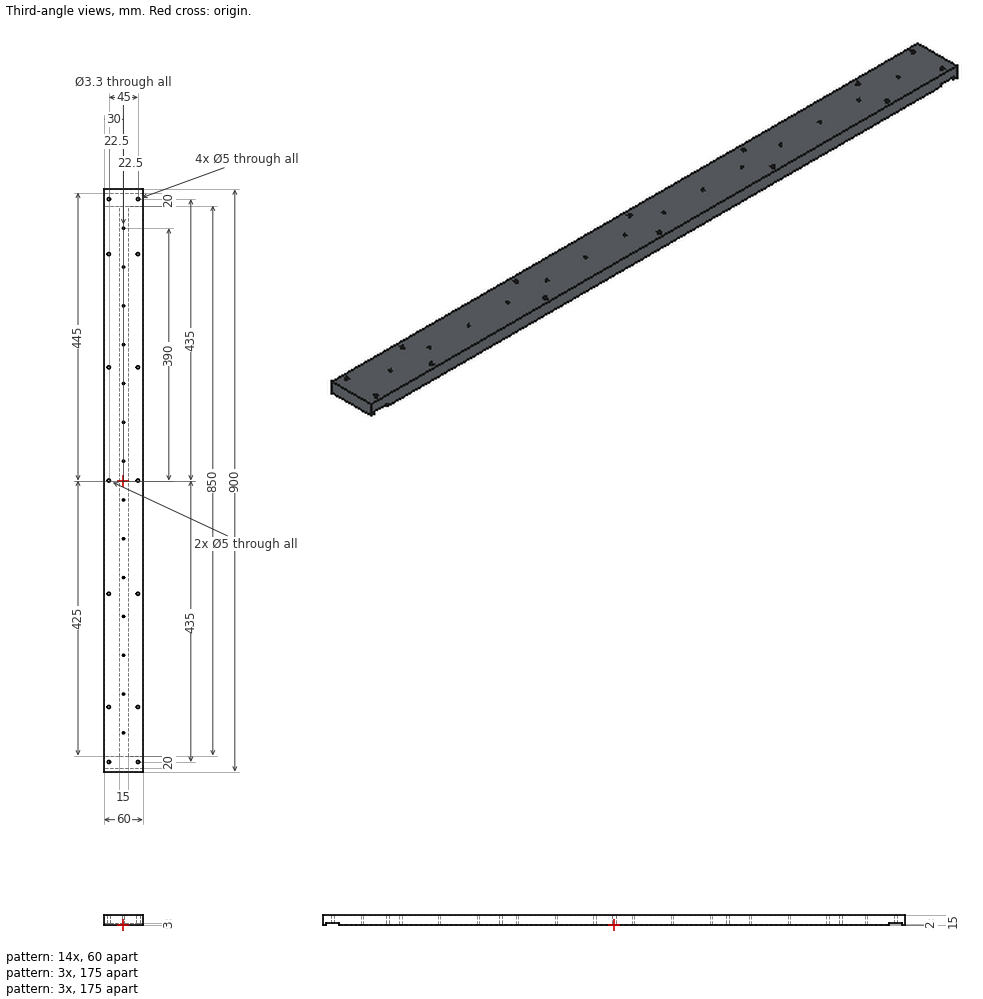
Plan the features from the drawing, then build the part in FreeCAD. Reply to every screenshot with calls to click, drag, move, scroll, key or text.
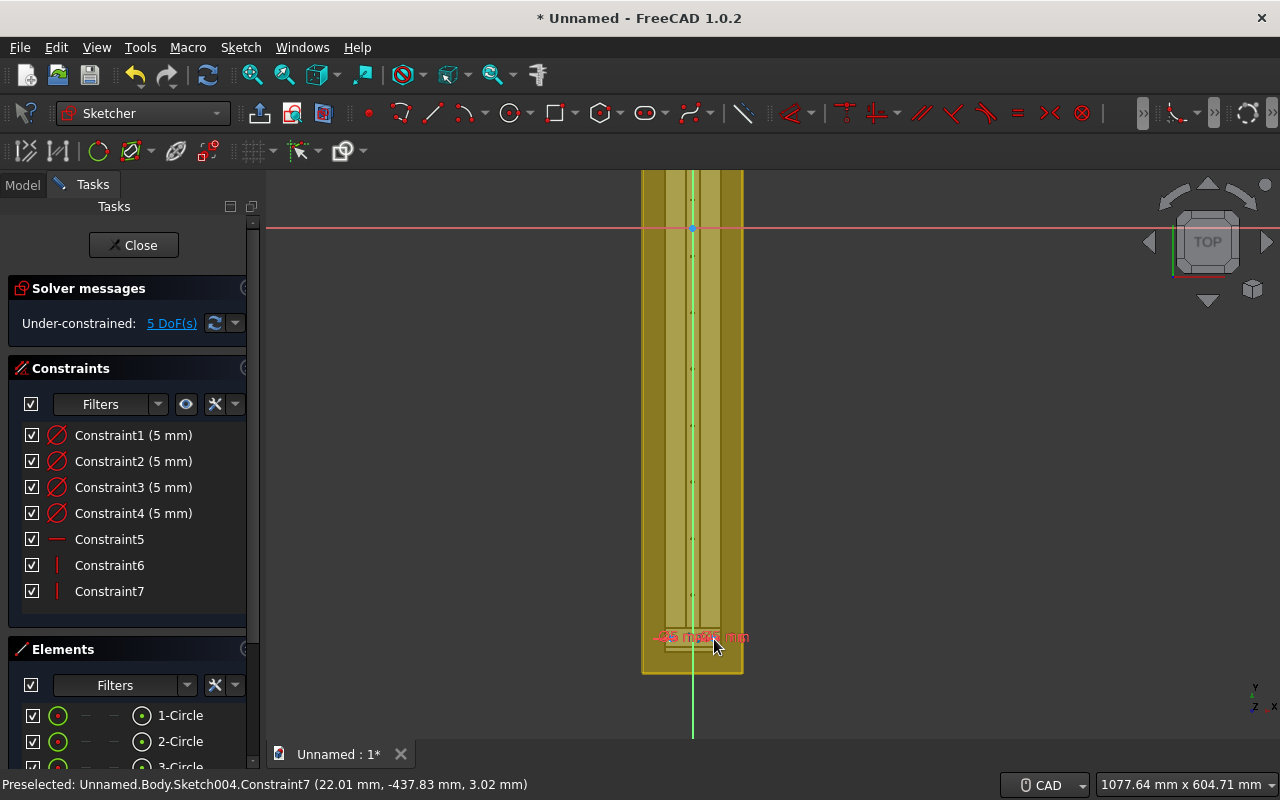
click(713, 639)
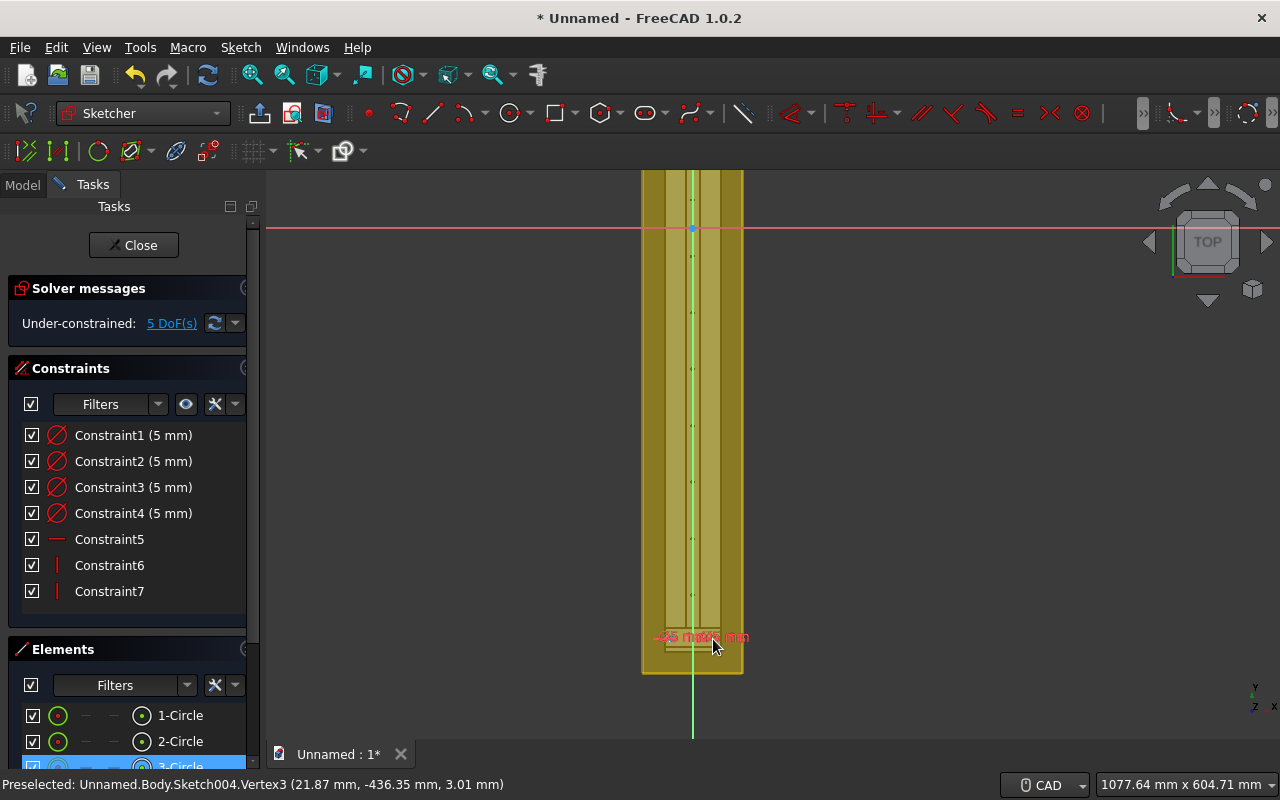
click(671, 639)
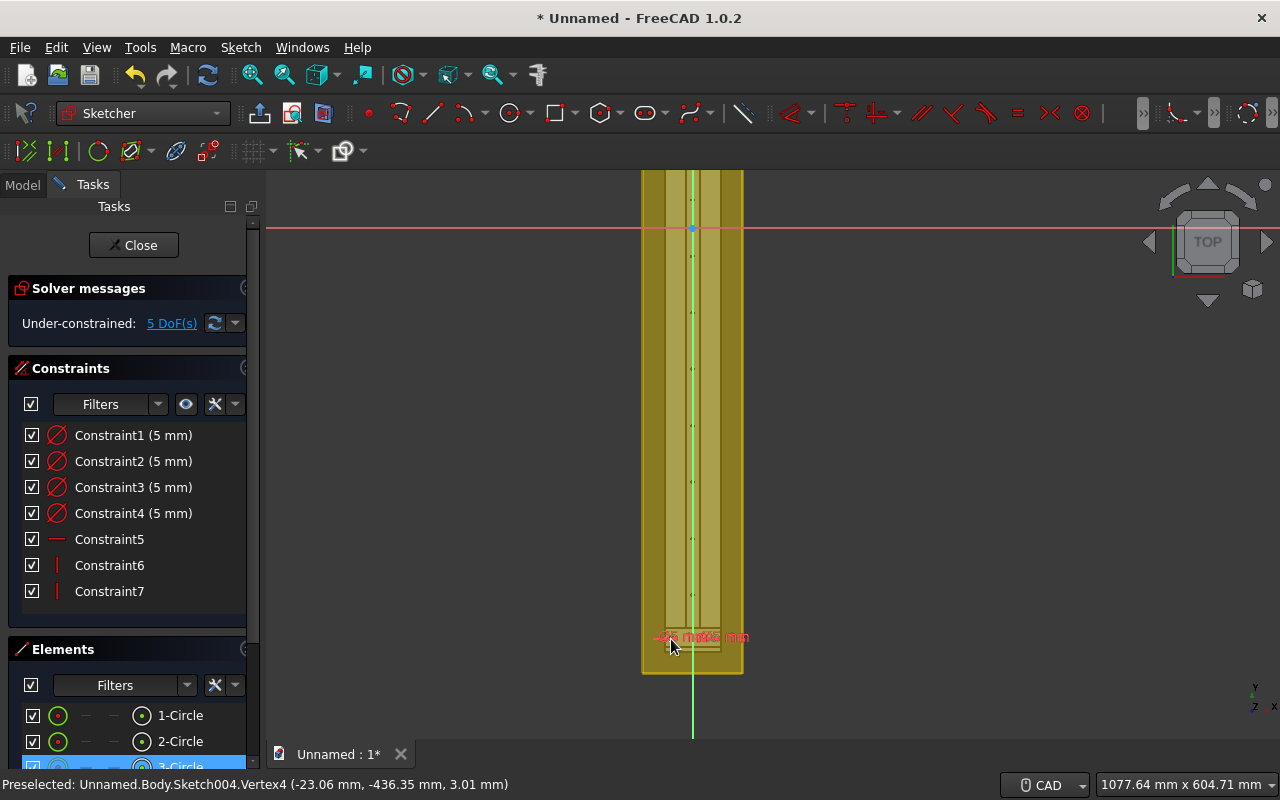
click(900, 114)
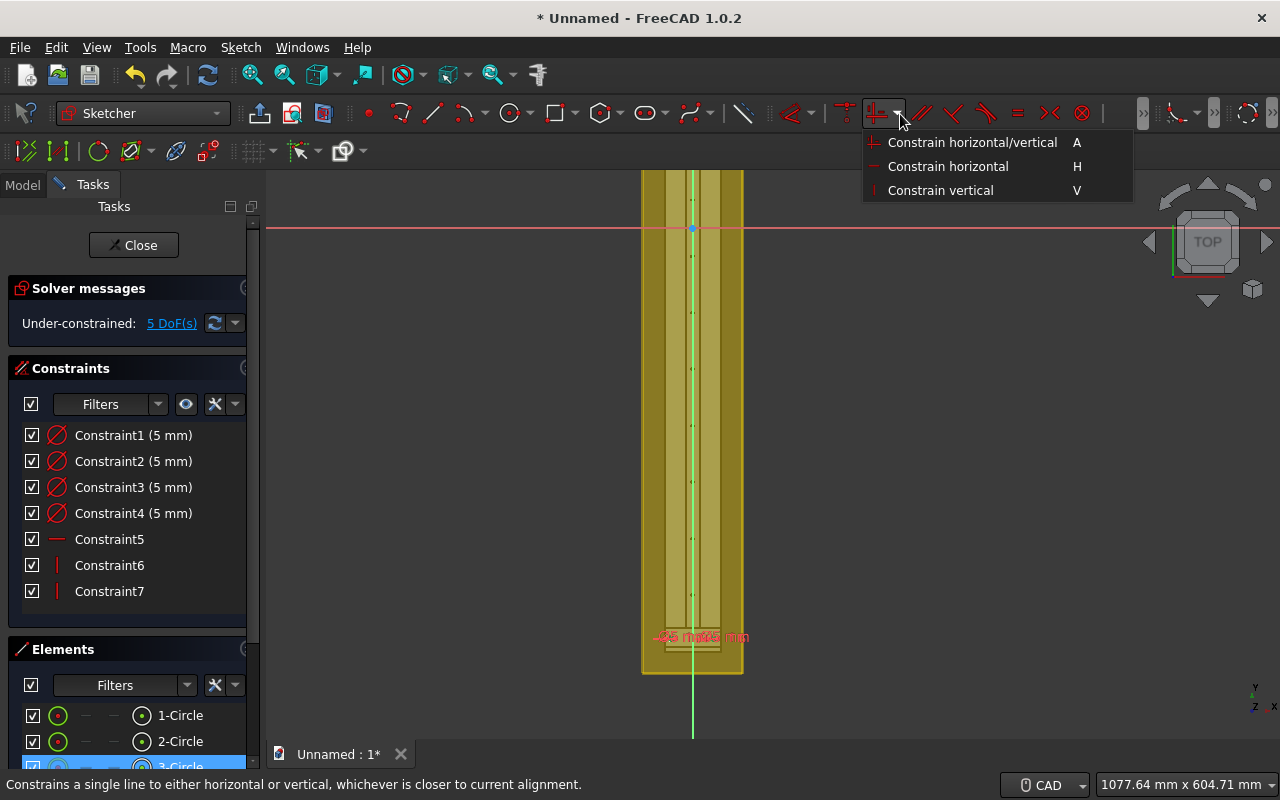
click(998, 166)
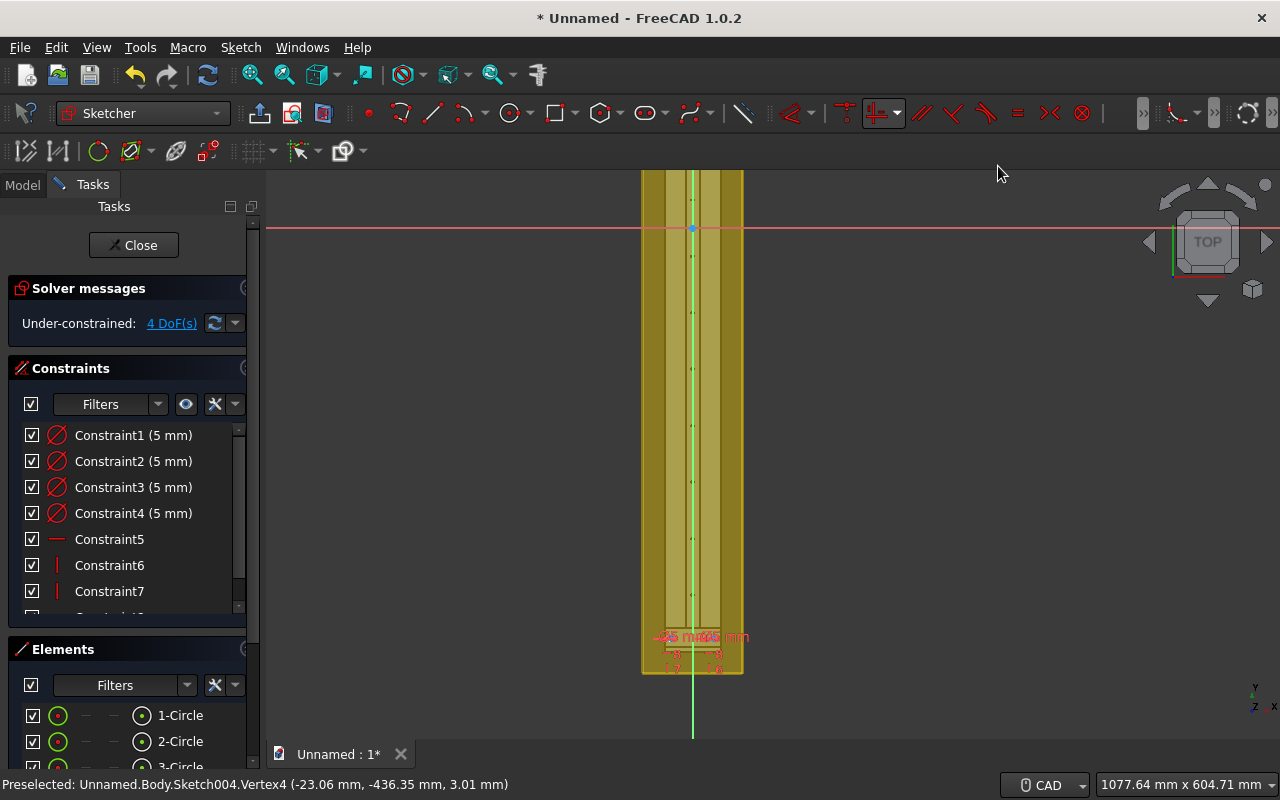
key(d)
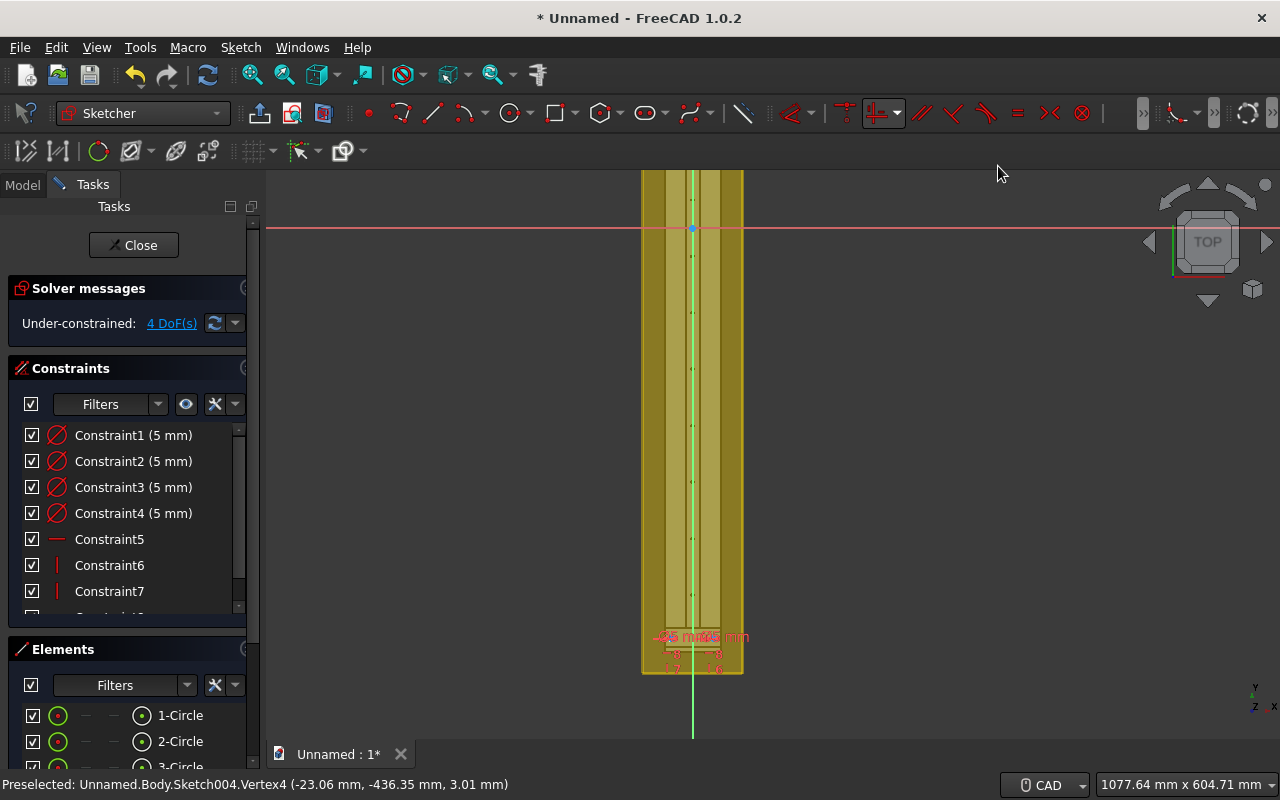
scroll(714, 639, down, 4)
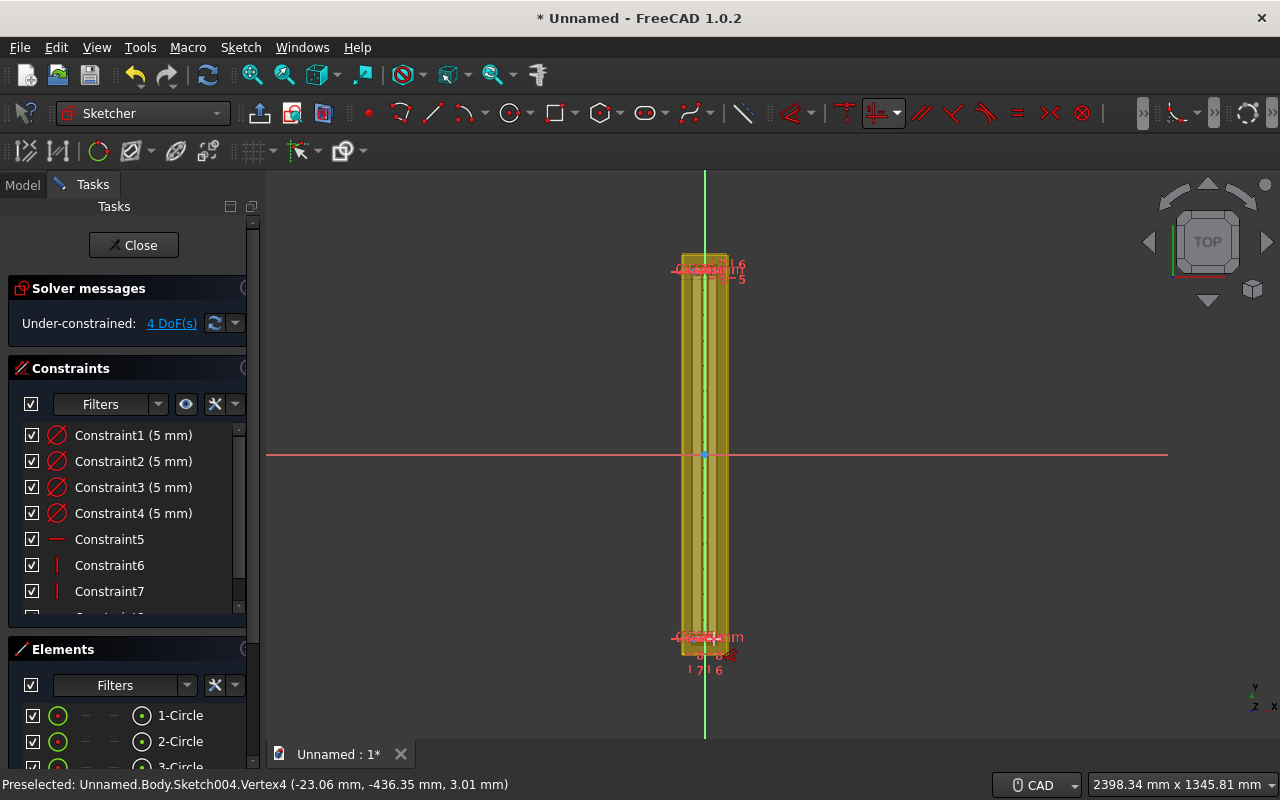
click(714, 272)
click(748, 363)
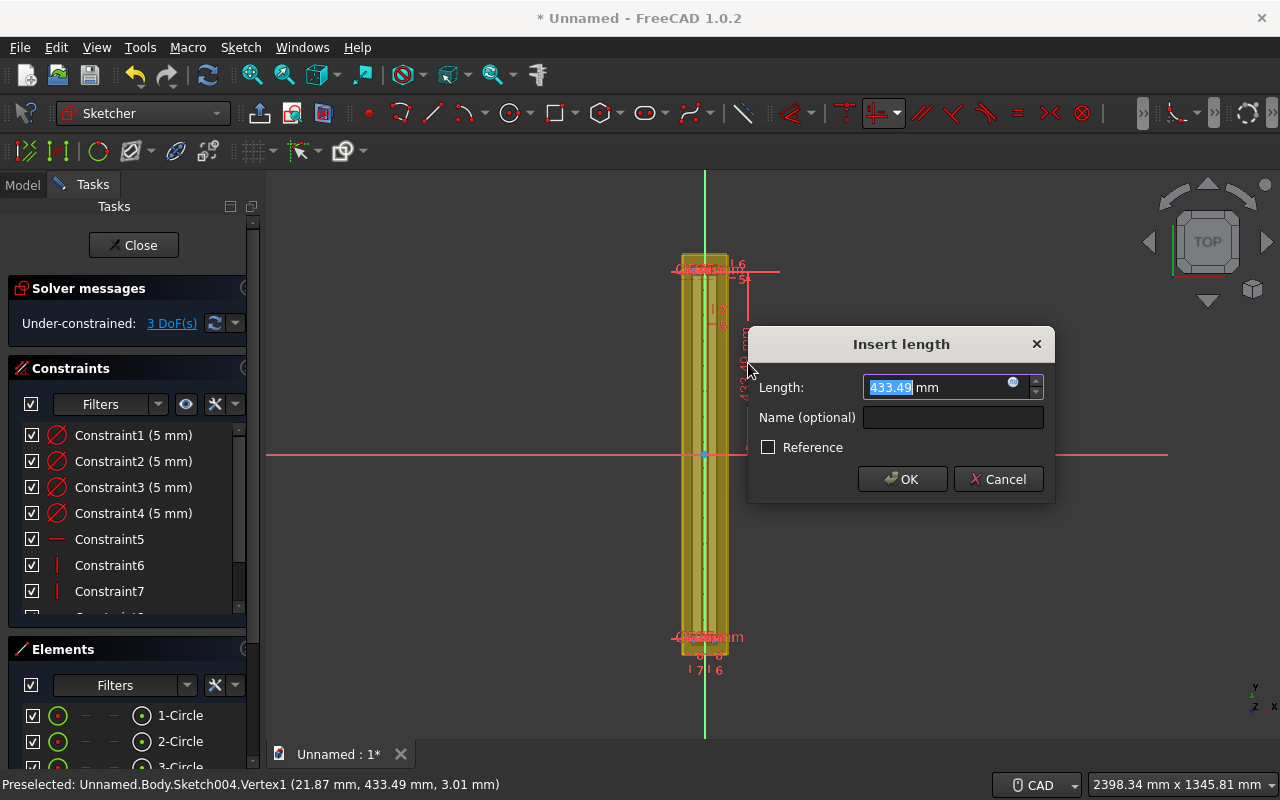
text(435)
key(Return)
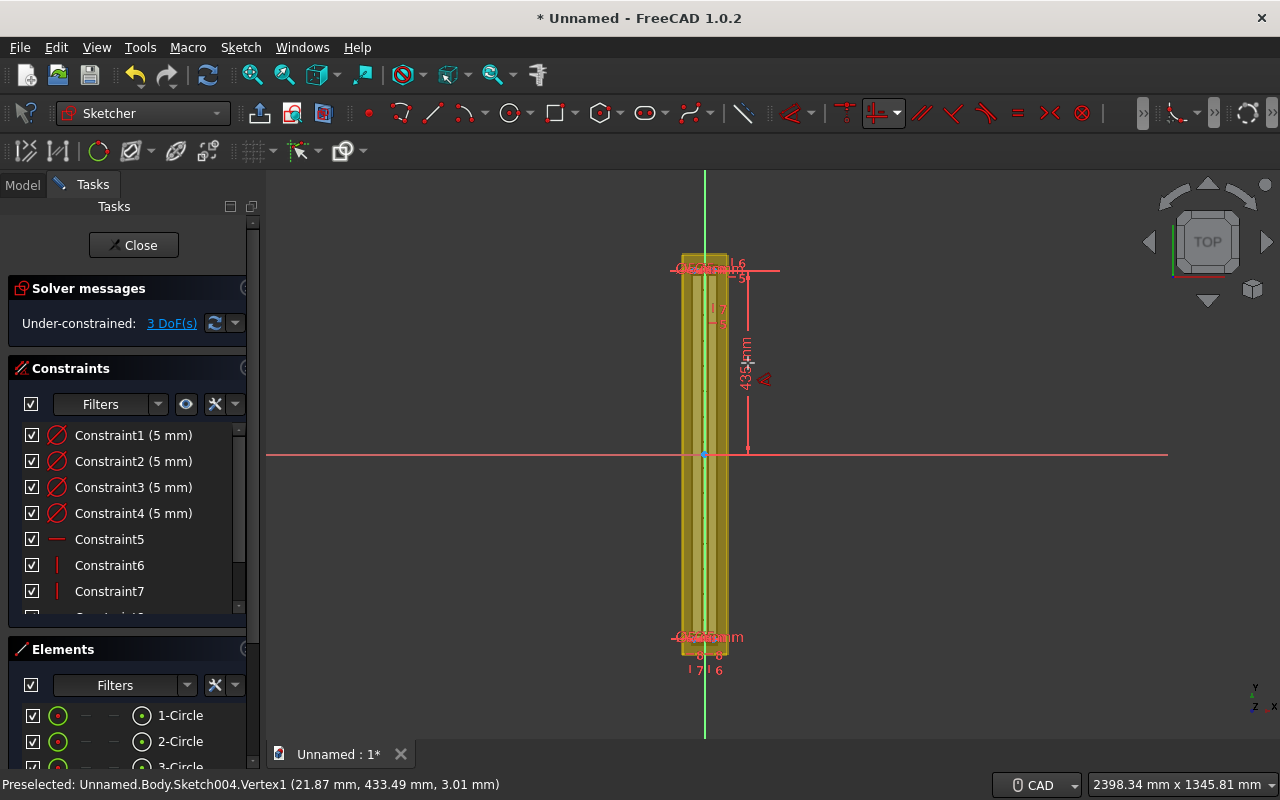
click(714, 639)
click(748, 547)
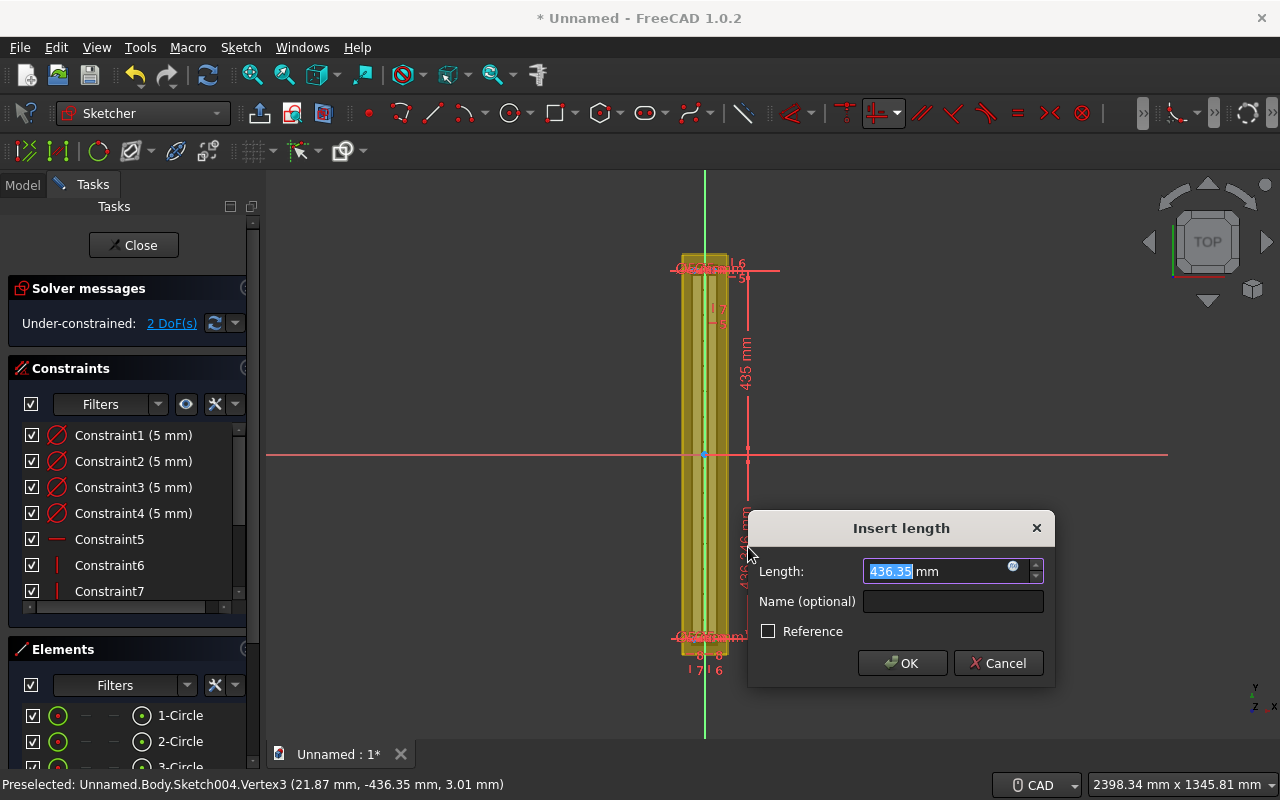
text(435)
key(Return)